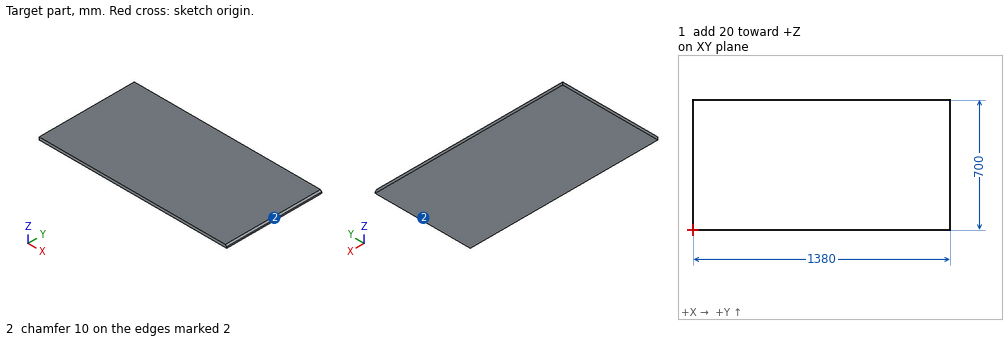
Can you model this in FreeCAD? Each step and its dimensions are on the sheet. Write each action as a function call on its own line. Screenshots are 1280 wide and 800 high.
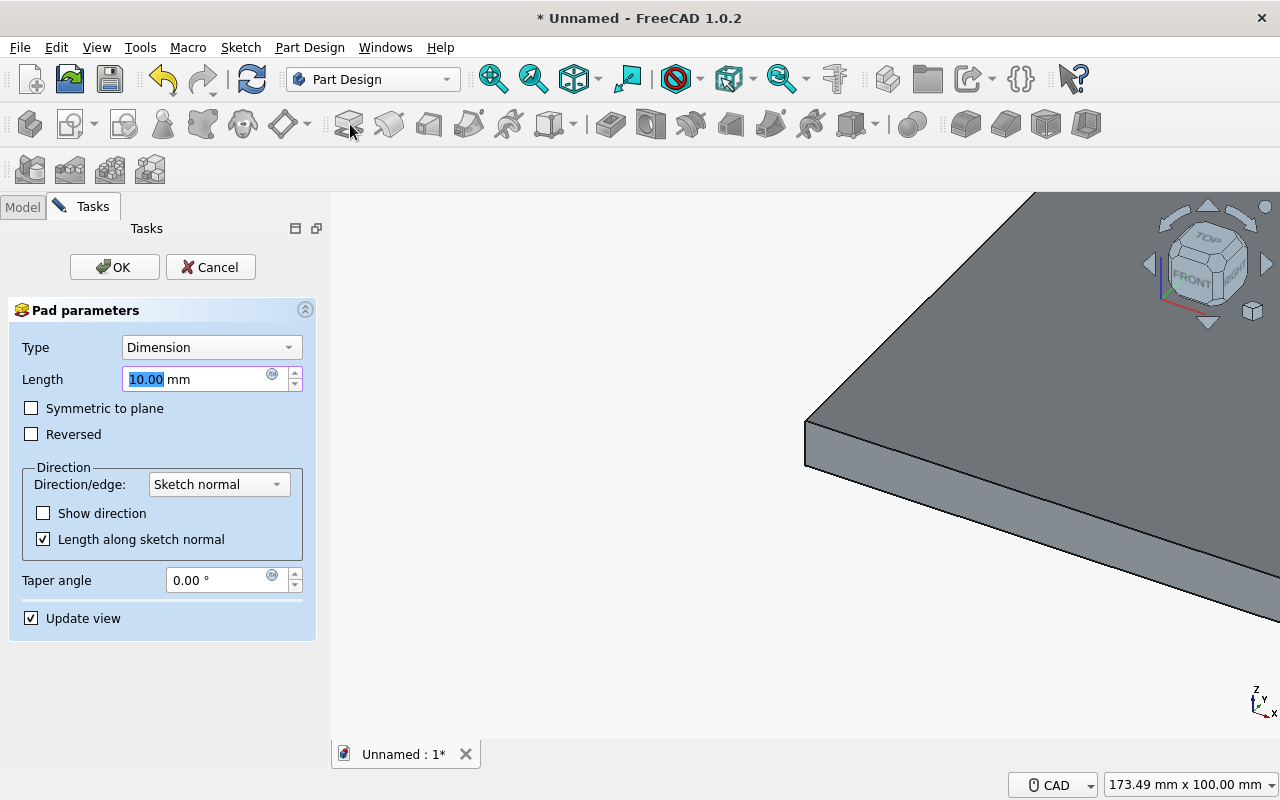
text(20)
key(Tab)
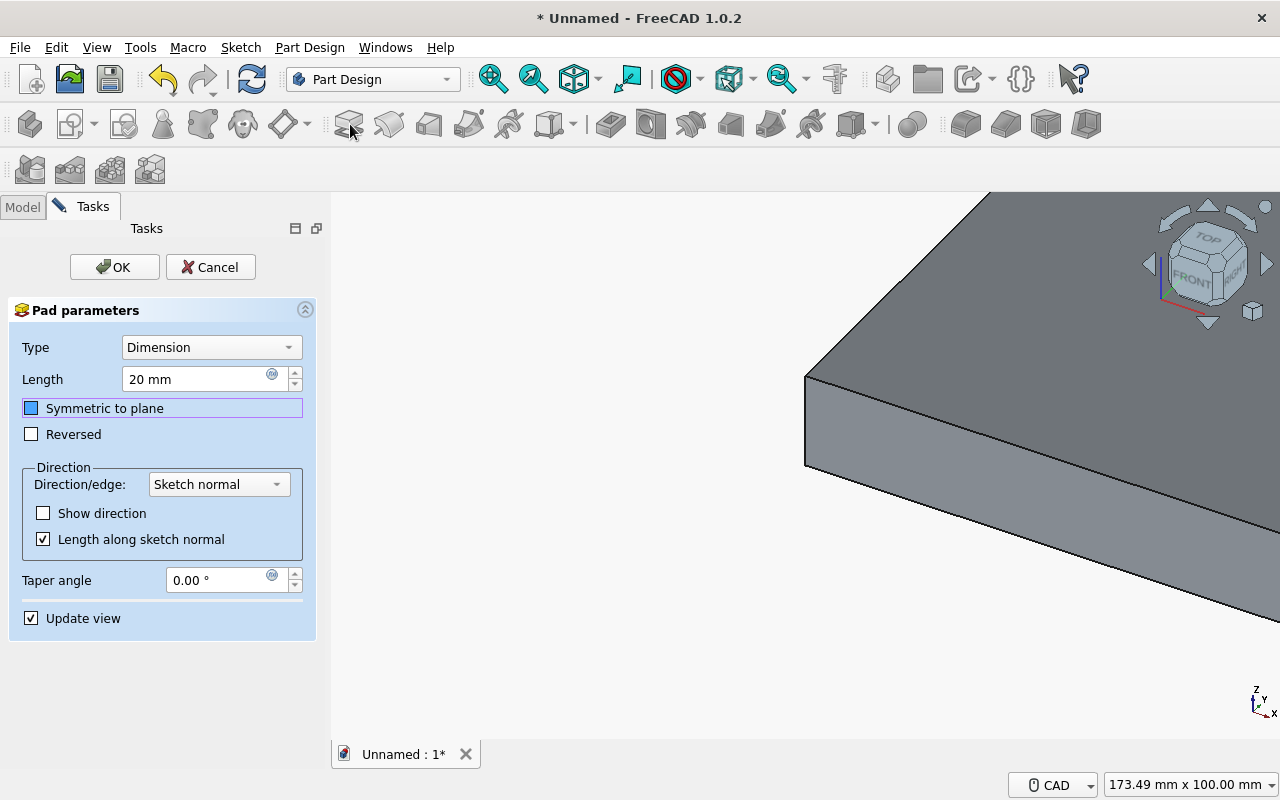
click(115, 267)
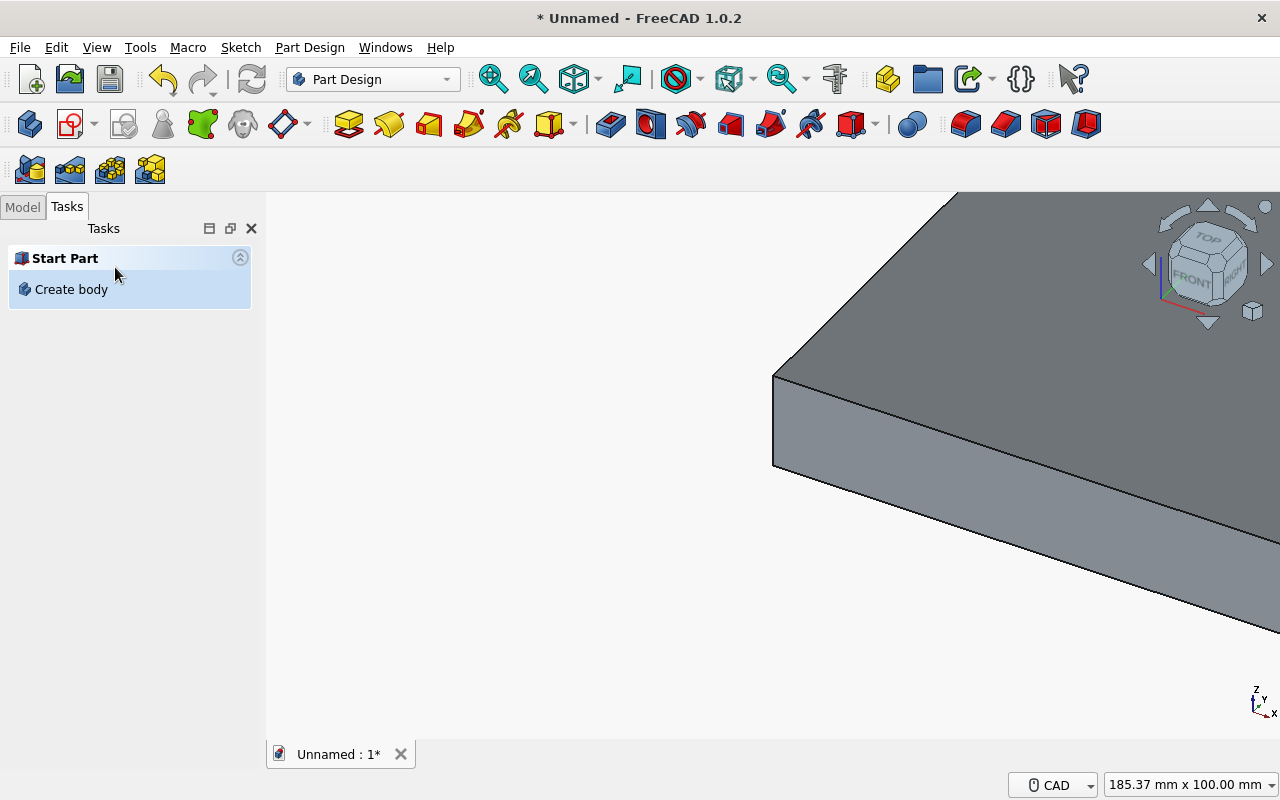
click(494, 80)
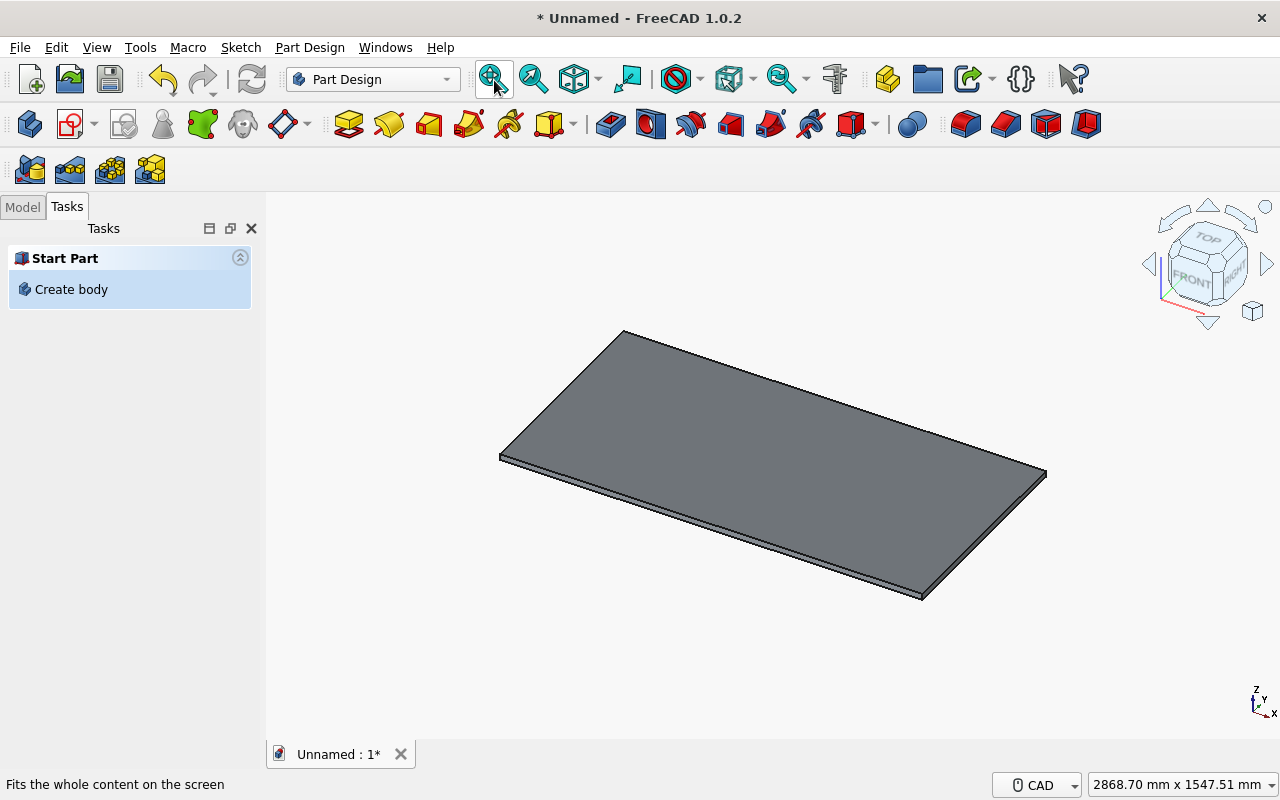
click(984, 532)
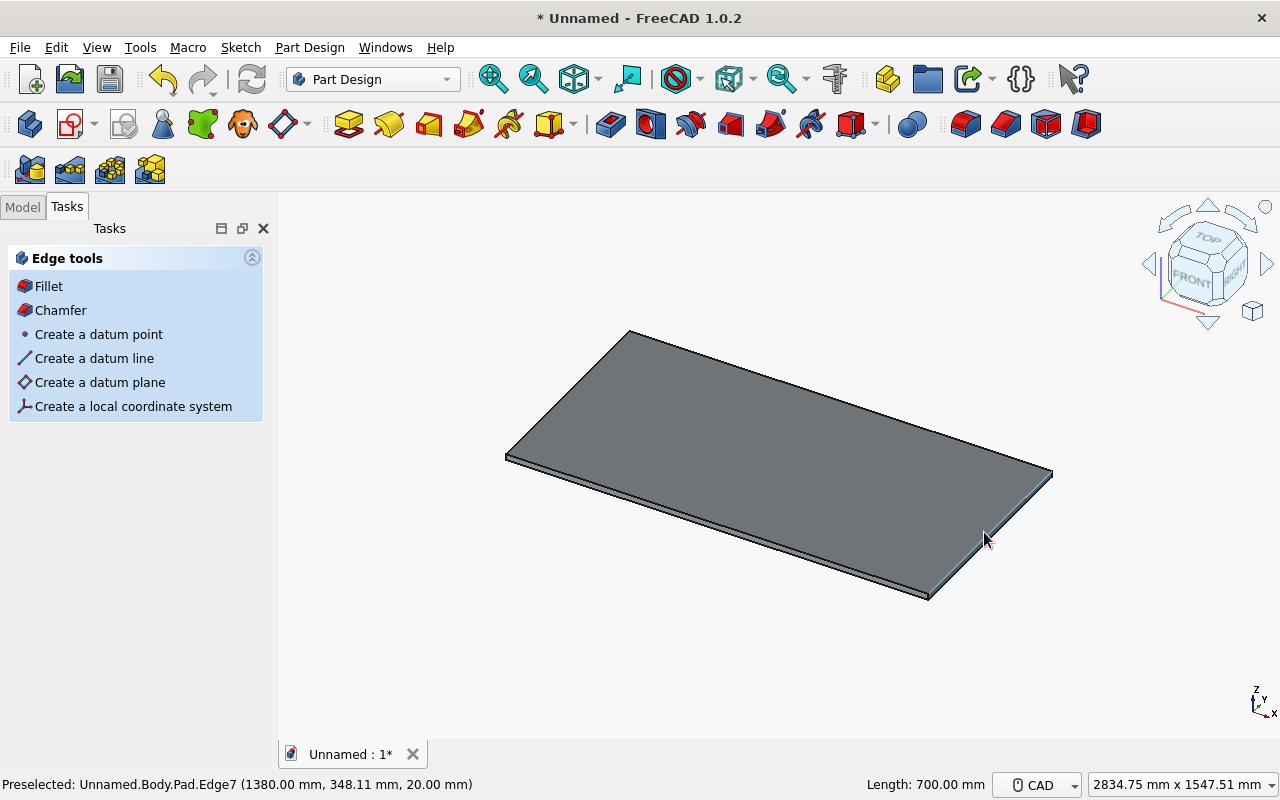
click(1006, 124)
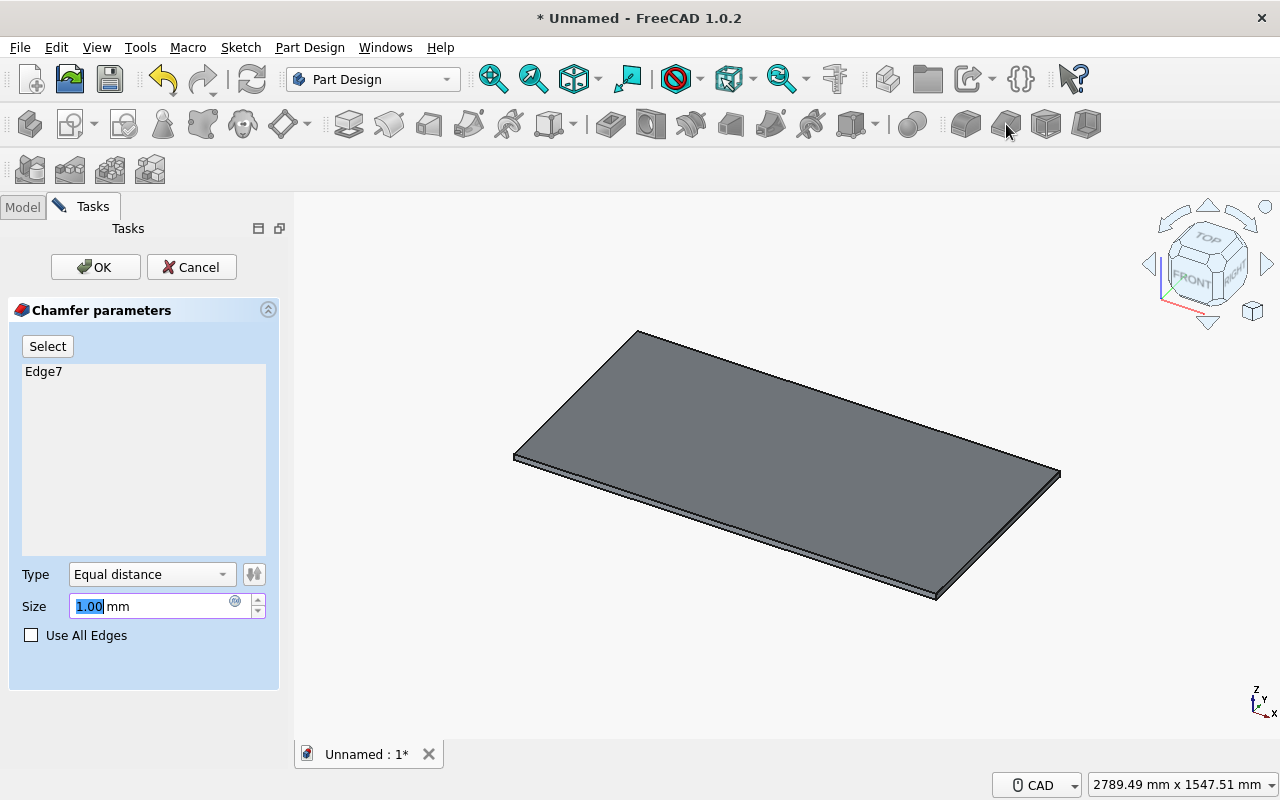
text(10)
key(Tab)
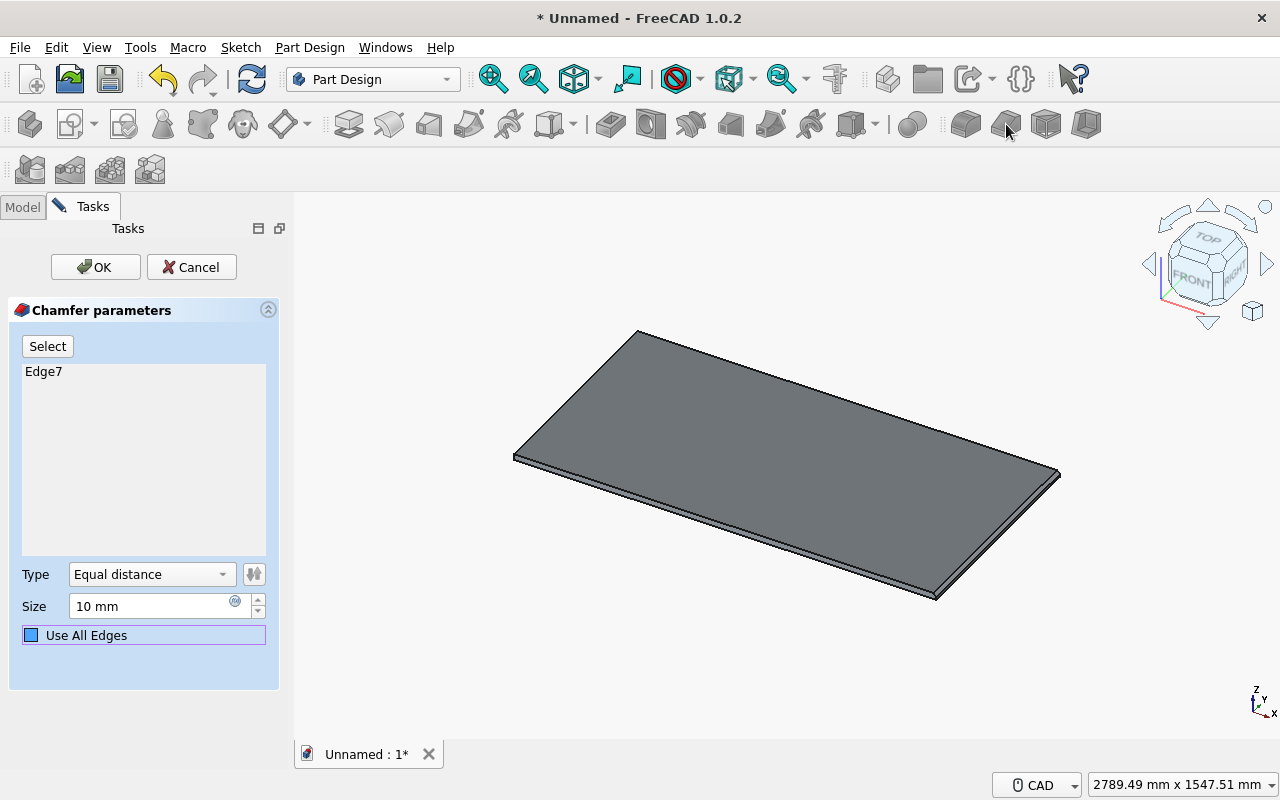
click(96, 267)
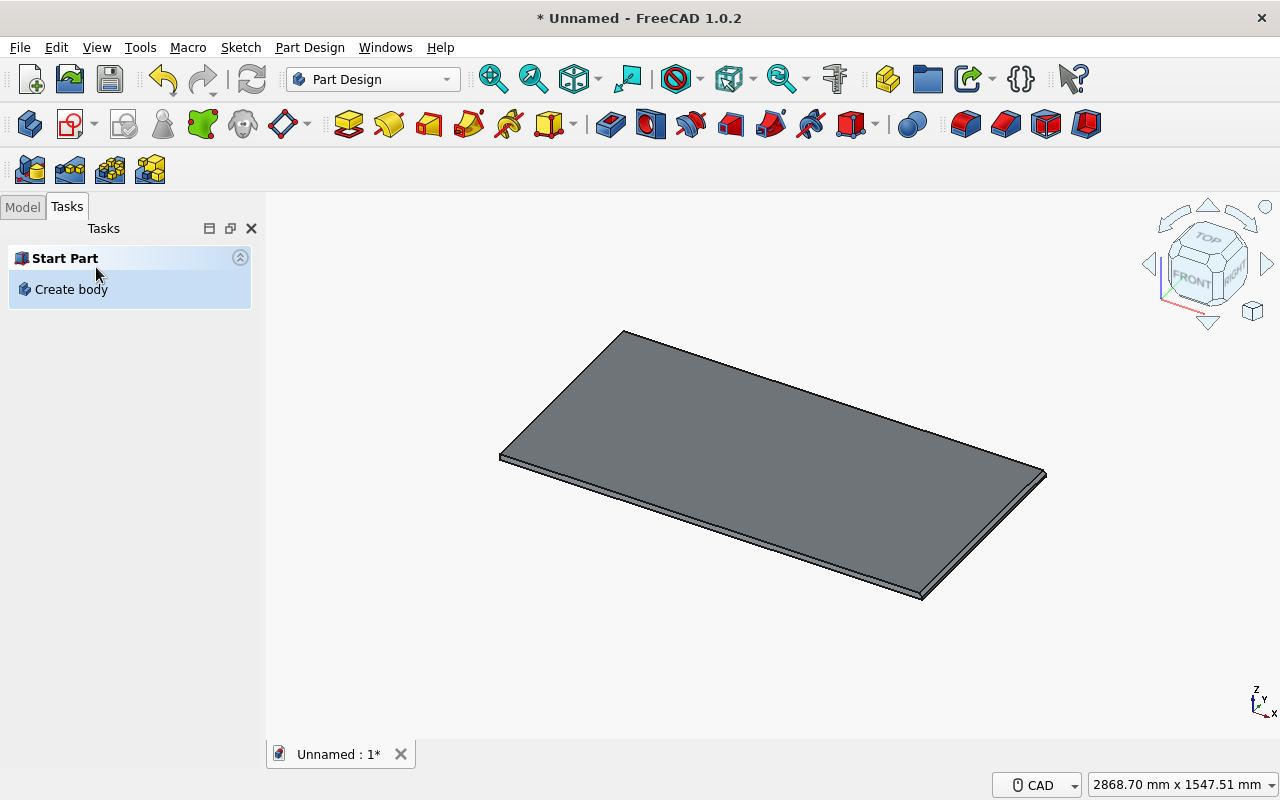
key(0)